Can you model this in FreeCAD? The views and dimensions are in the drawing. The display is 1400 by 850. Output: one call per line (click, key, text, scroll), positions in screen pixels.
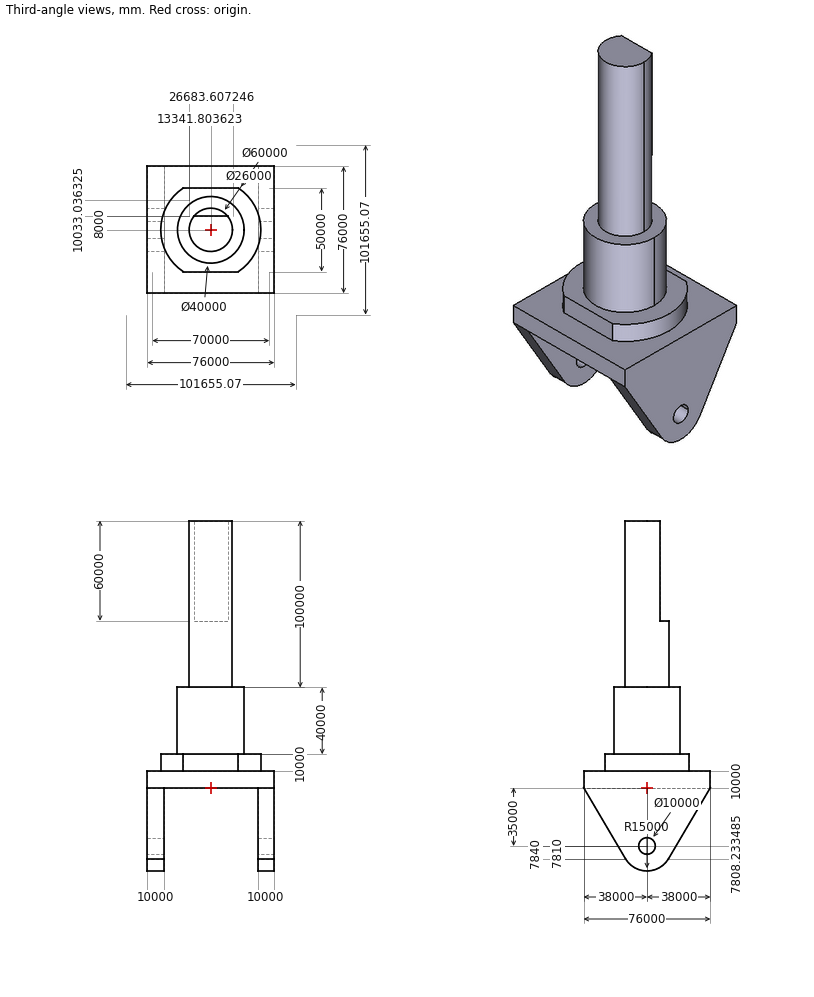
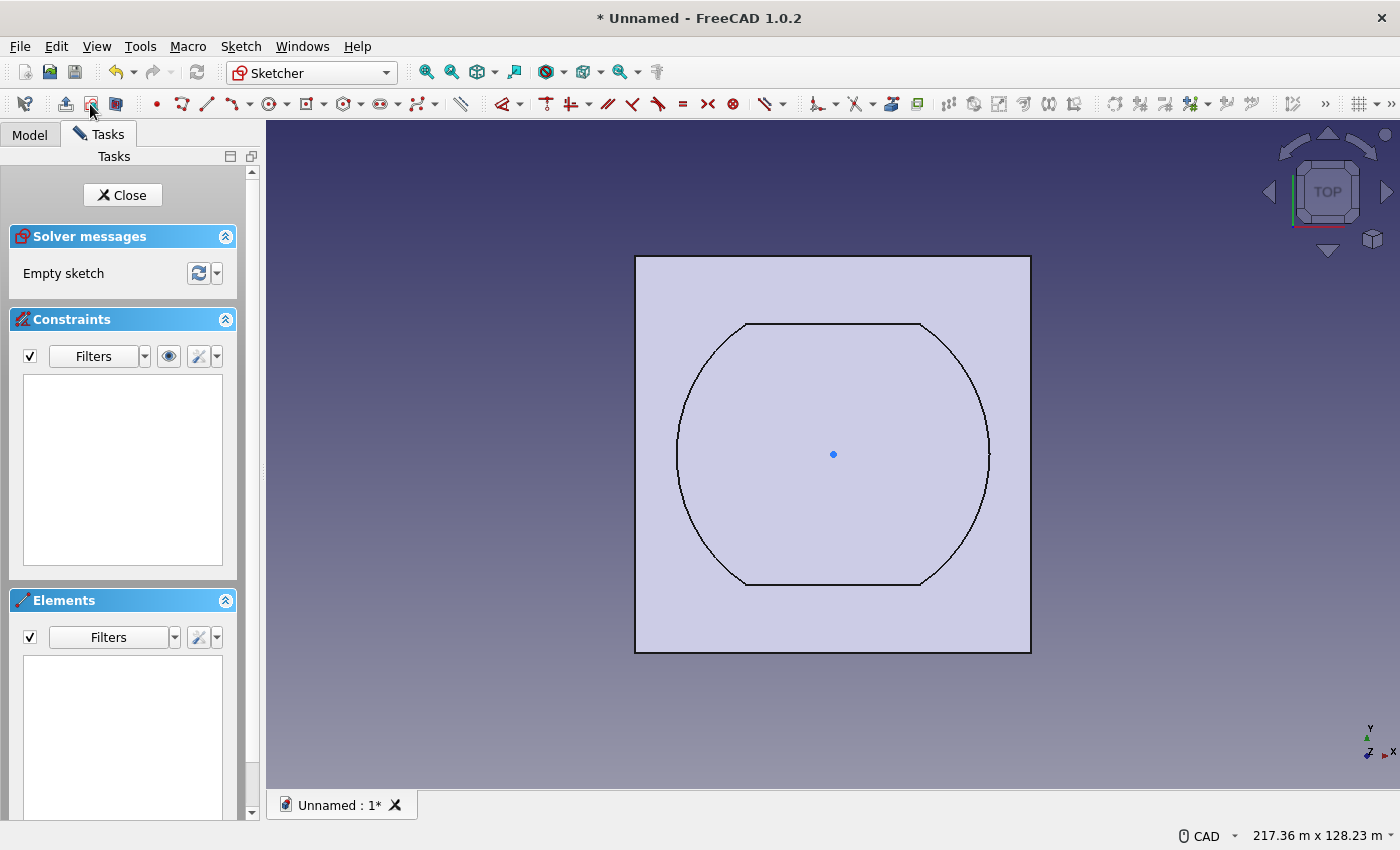
scroll(889, 455, up, 4)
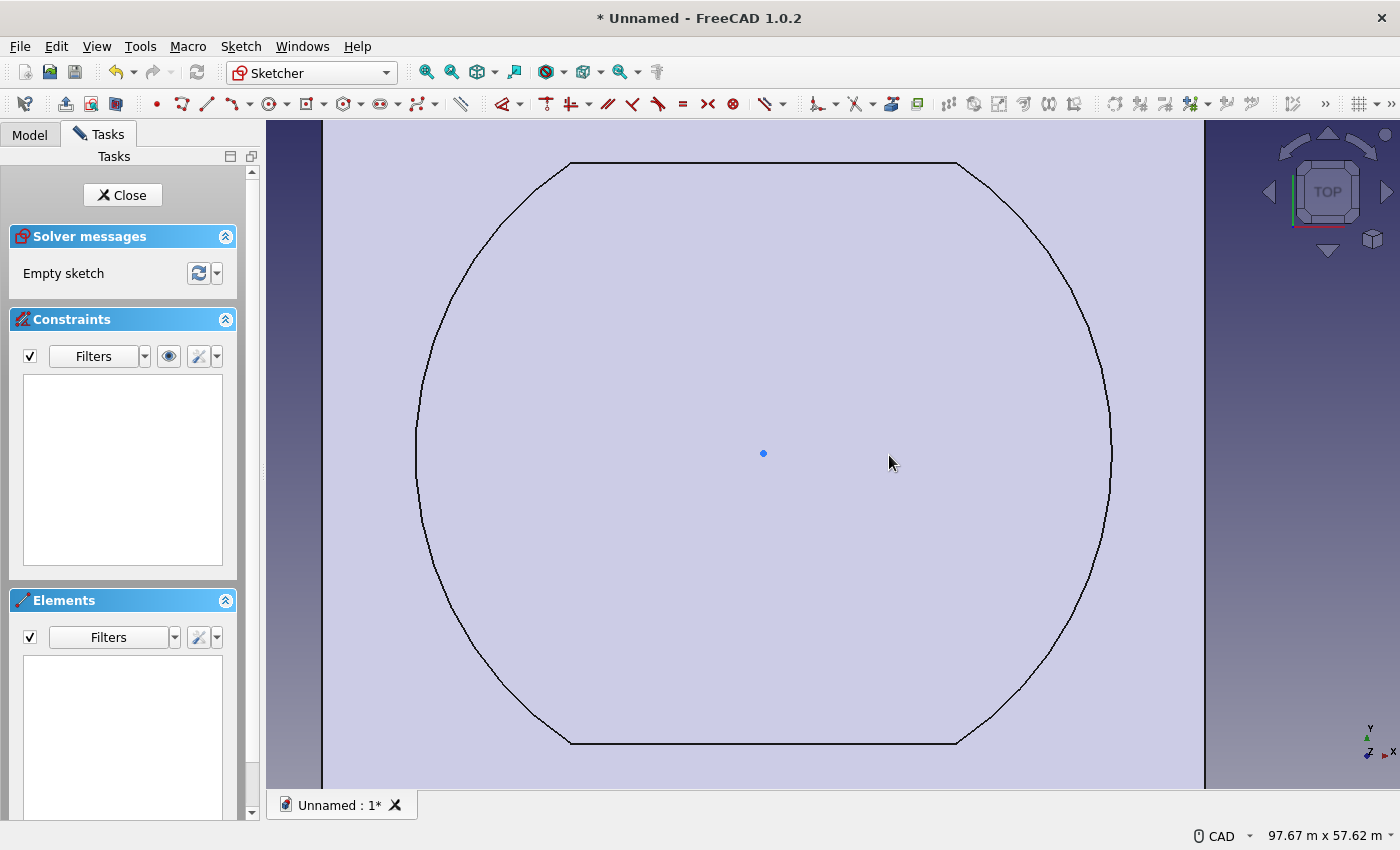
key(g)
key(c)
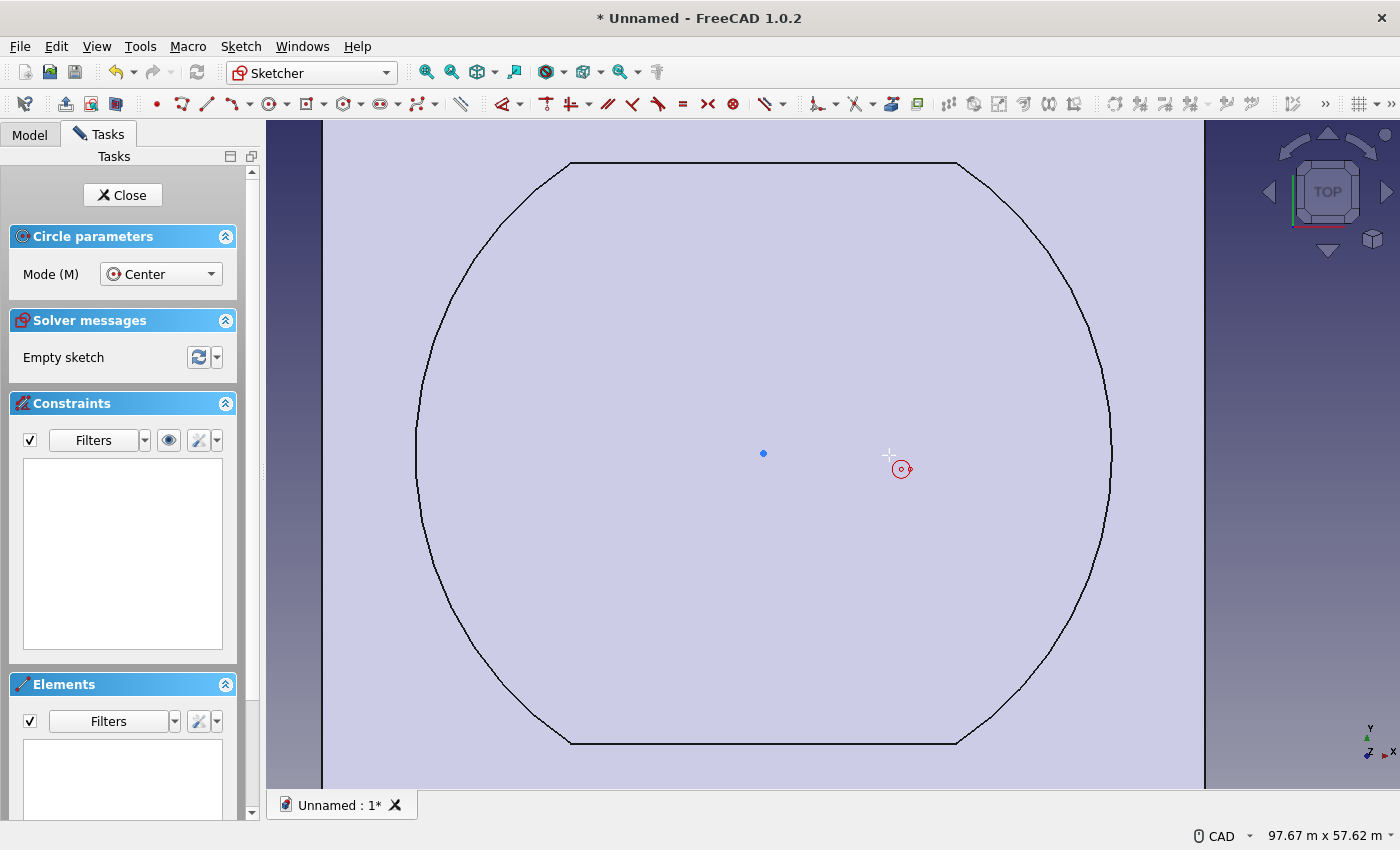
click(764, 453)
click(928, 289)
key(Escape)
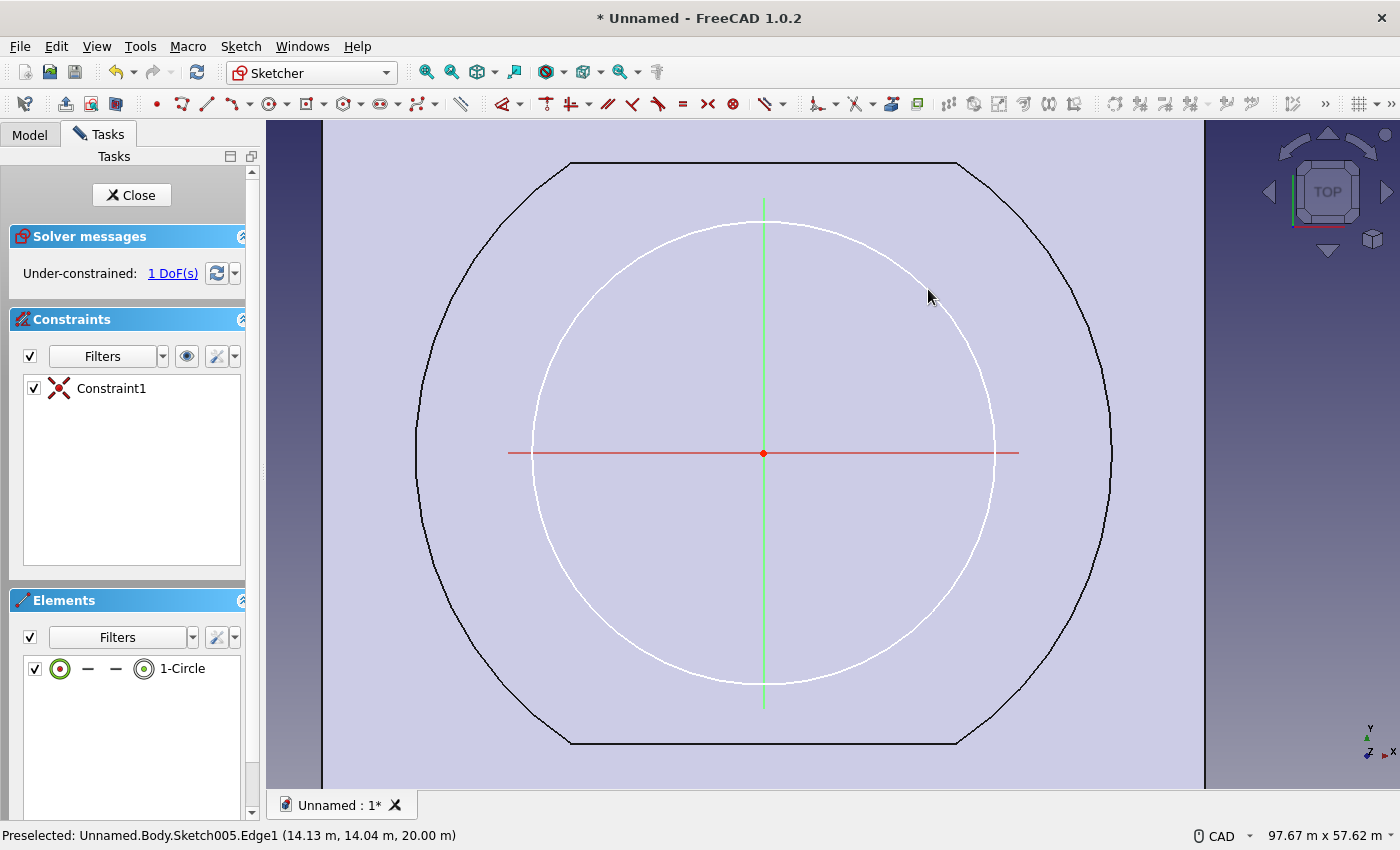
click(502, 104)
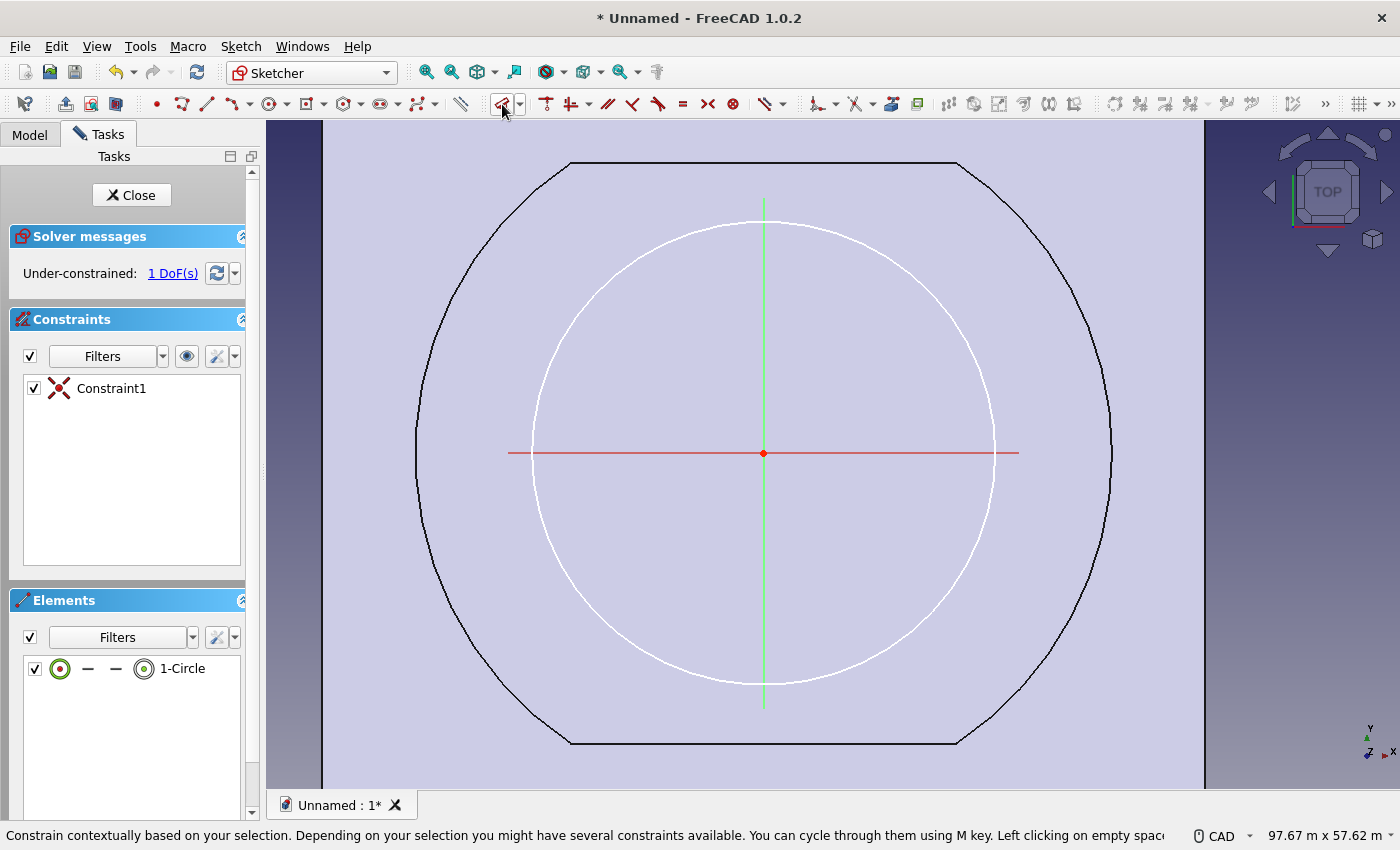
click(927, 289)
click(950, 266)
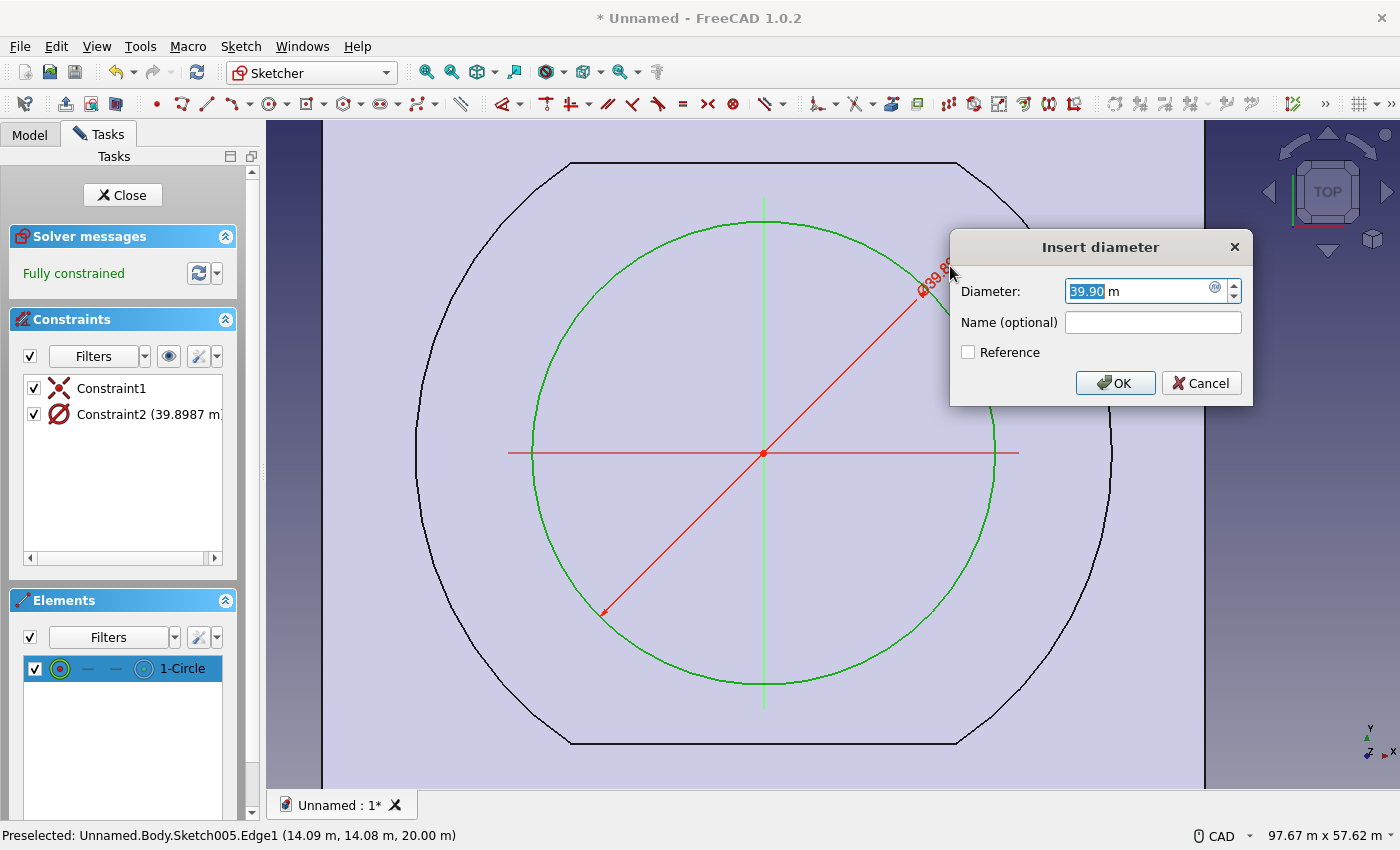
key(ctrl+a)
text(40000 mm)
key(Return)
key(Escape)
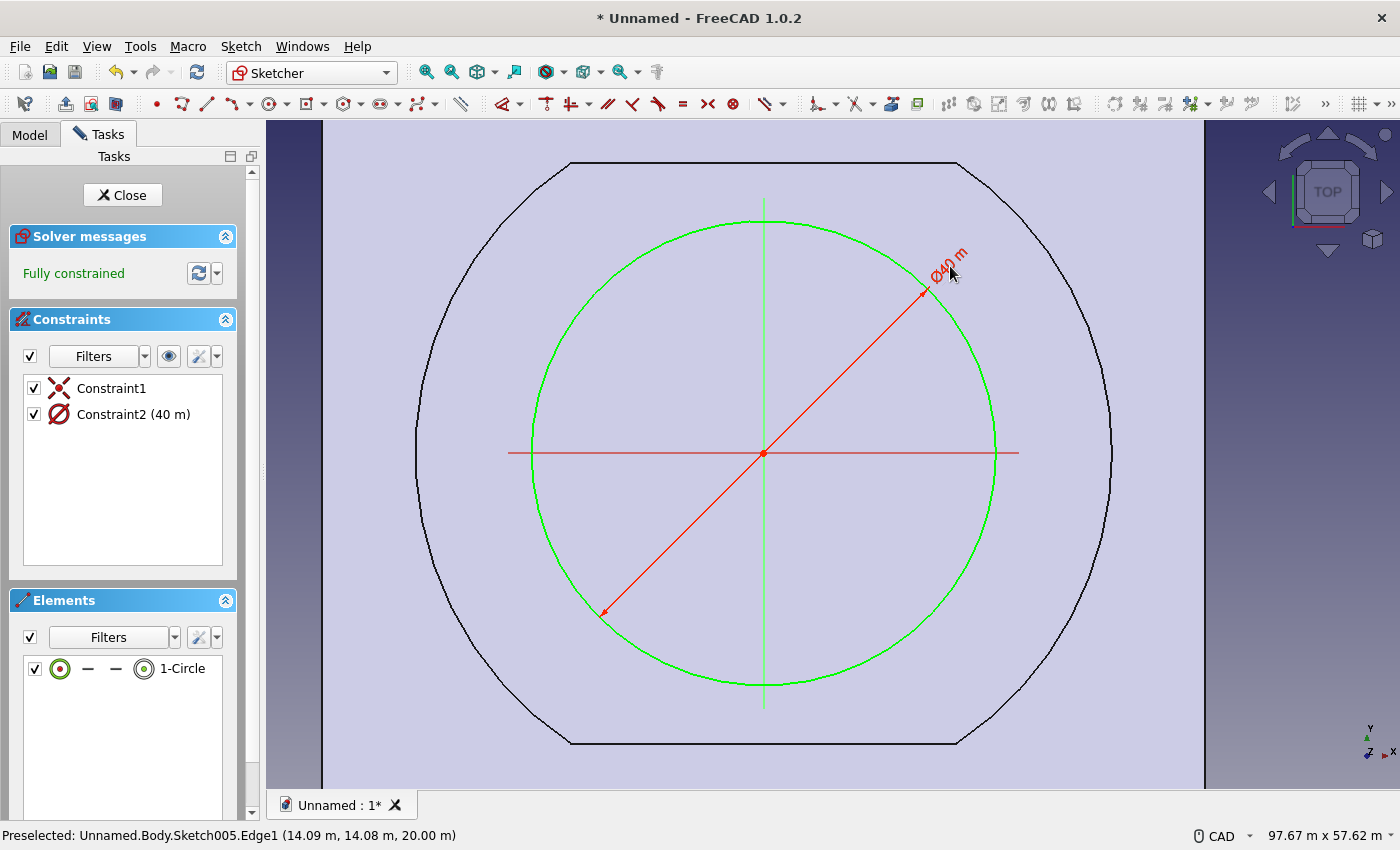
click(123, 195)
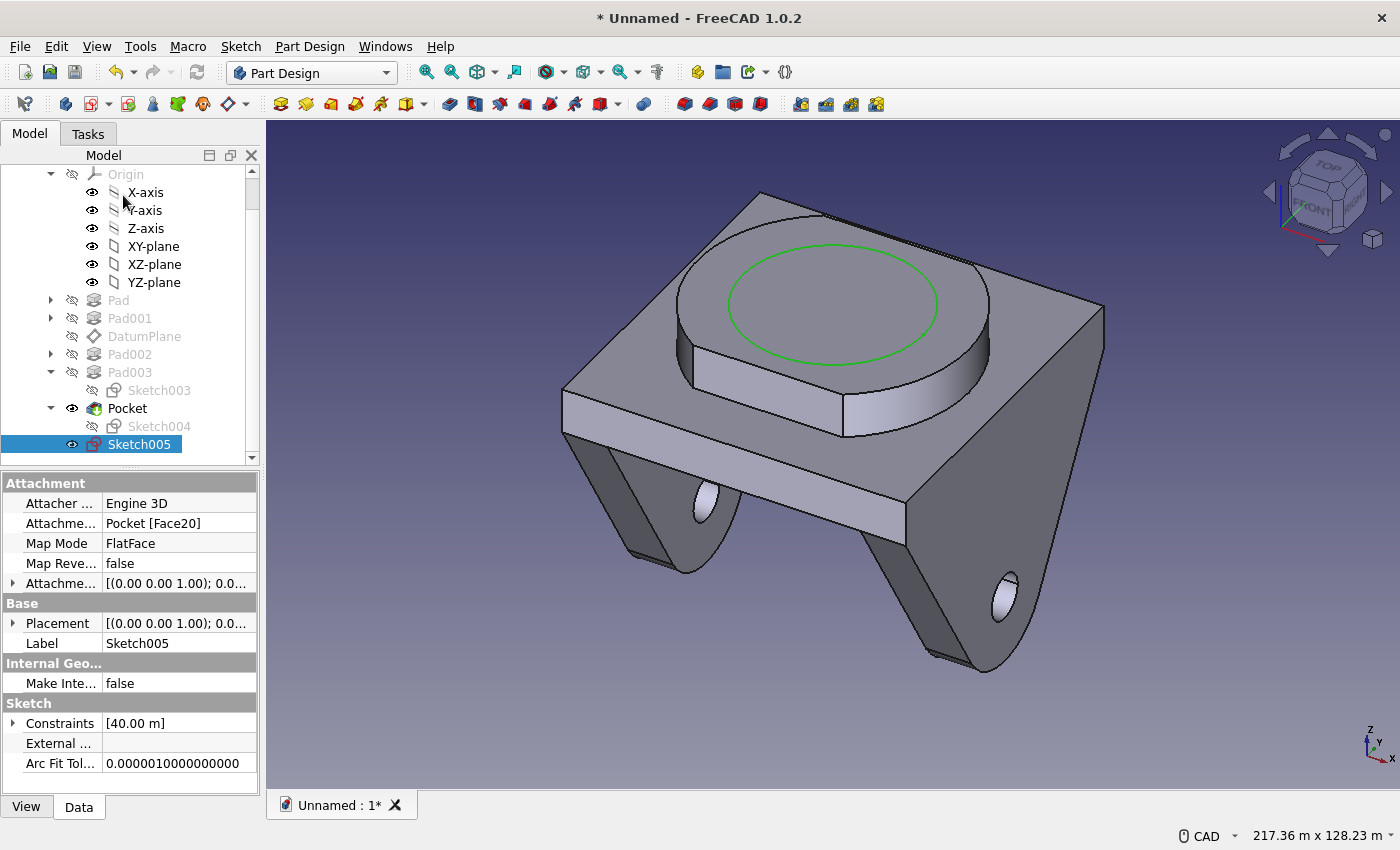
click(281, 104)